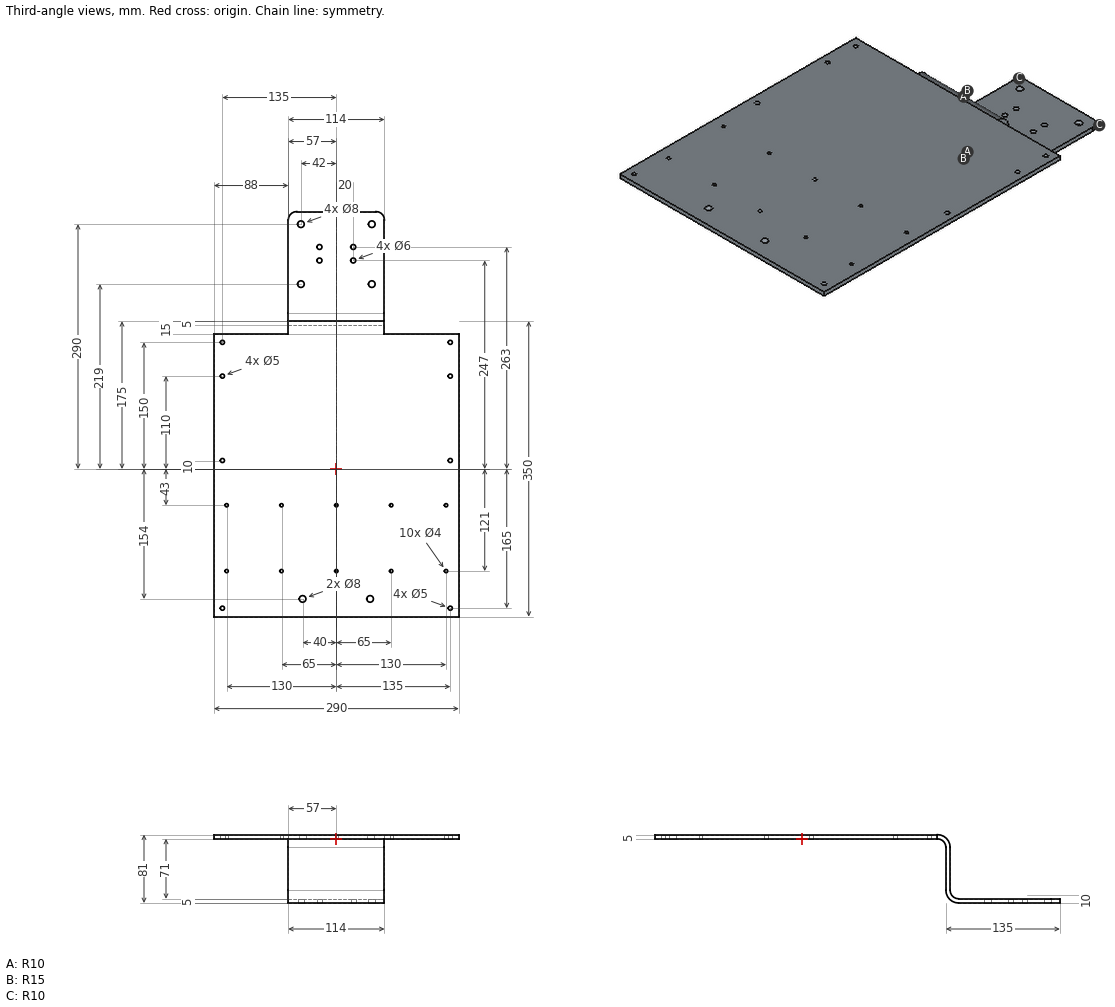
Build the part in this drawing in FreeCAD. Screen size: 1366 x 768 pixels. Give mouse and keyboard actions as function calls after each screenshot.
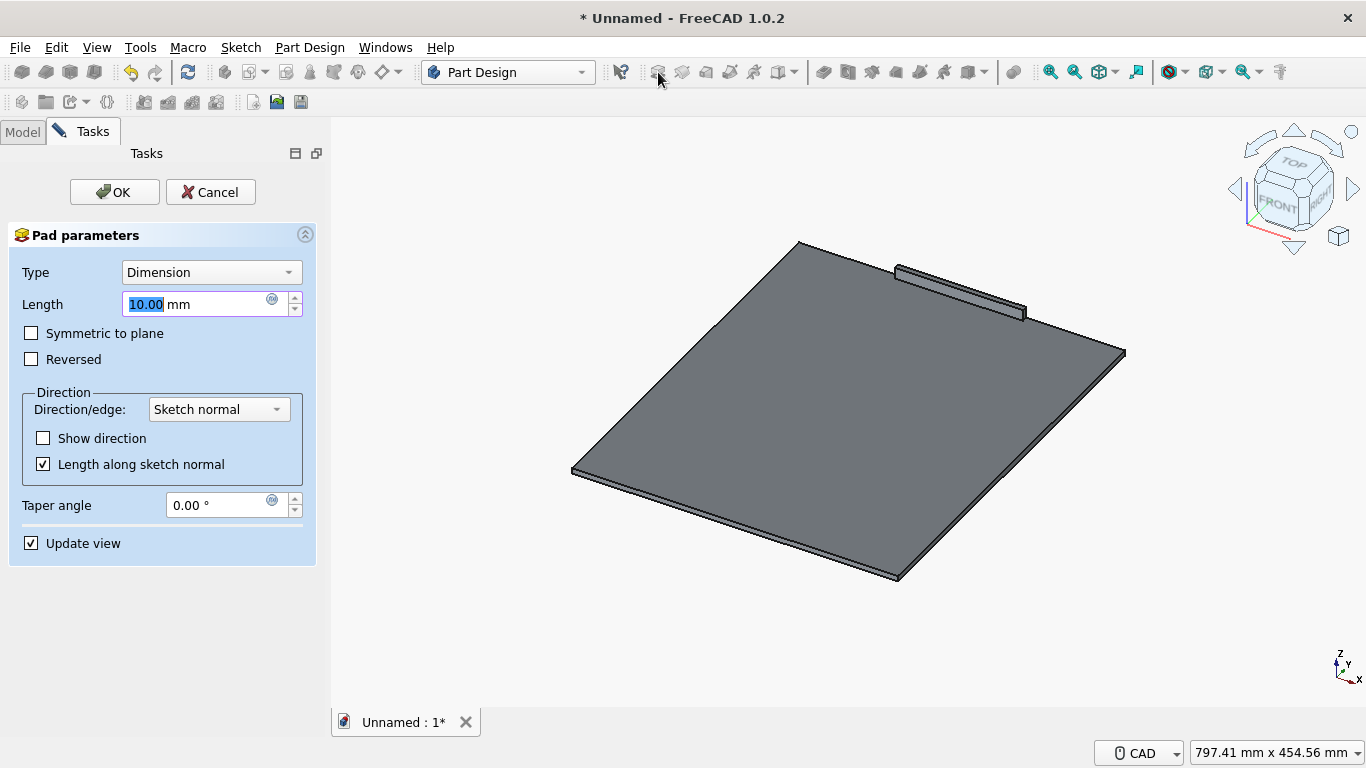
text(81)
key(Tab)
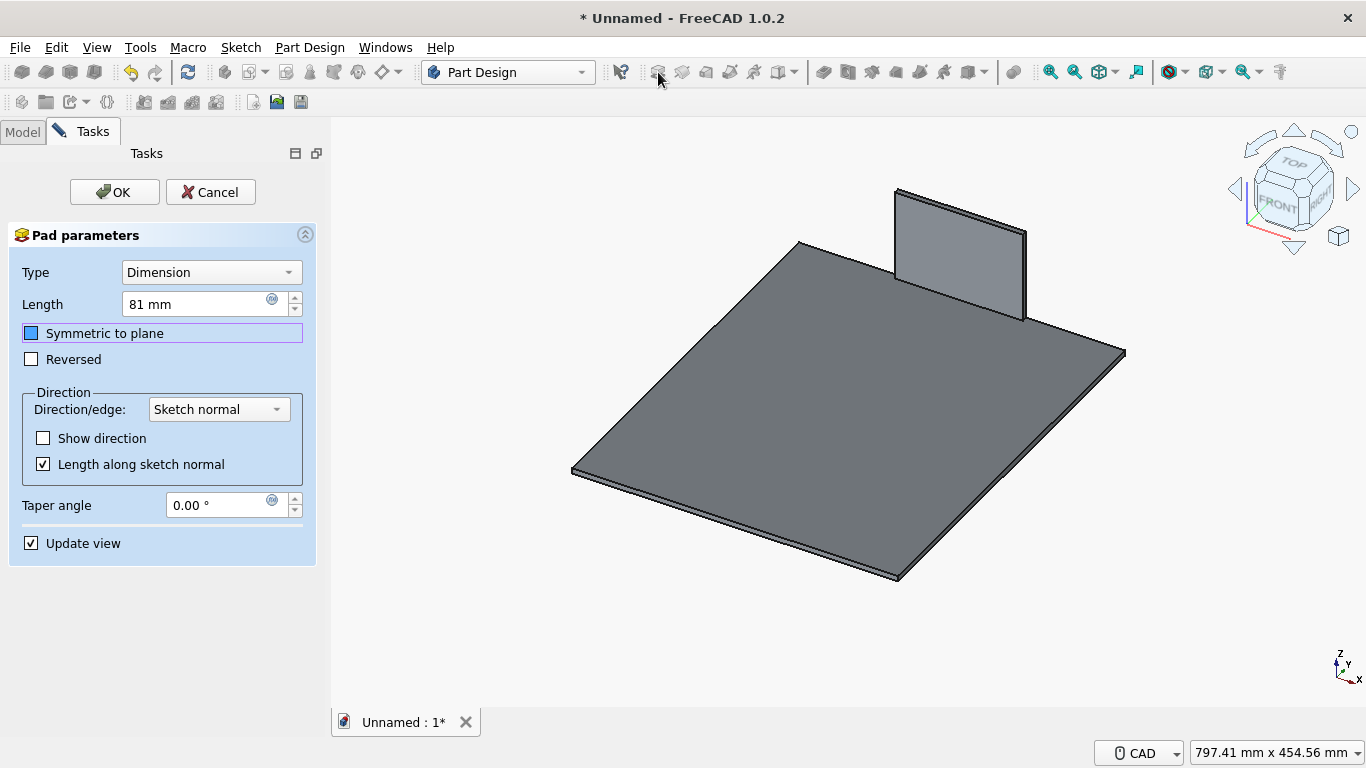
click(30, 359)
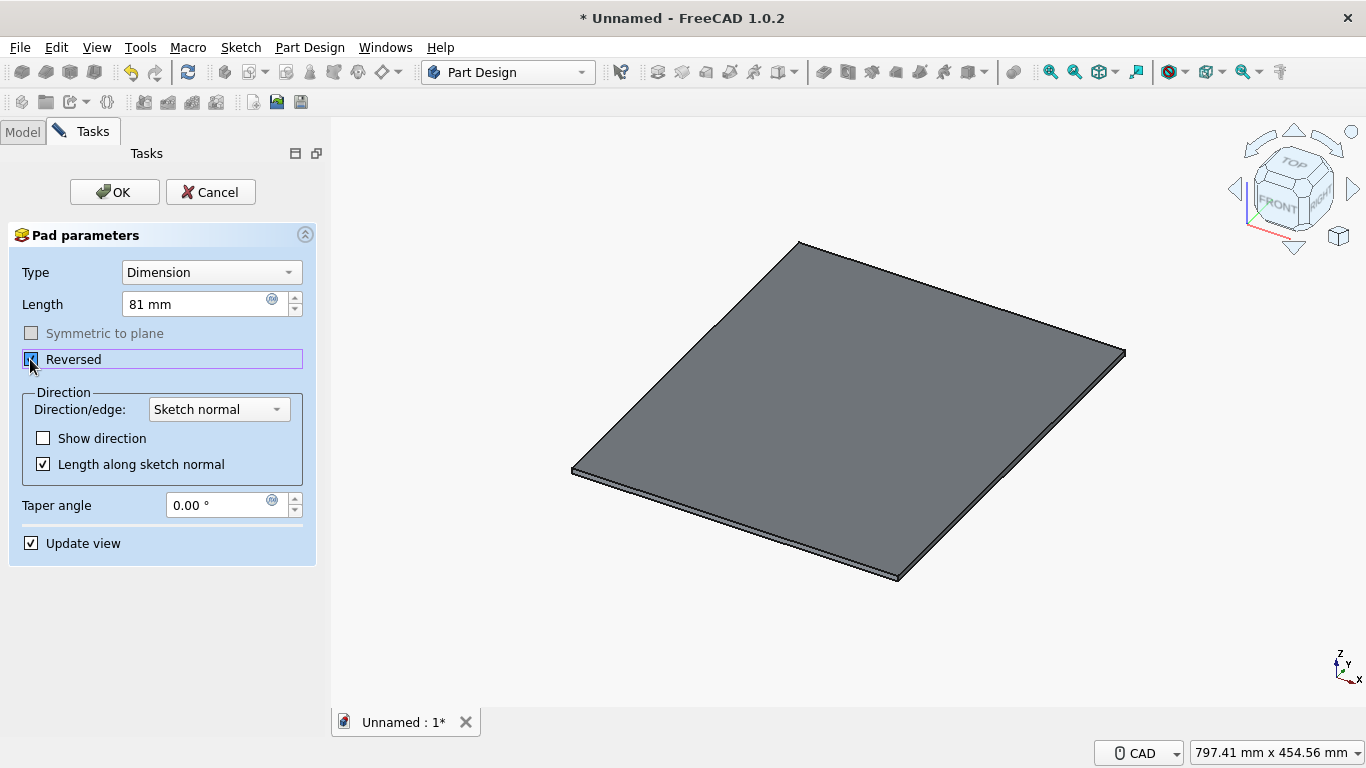
click(115, 192)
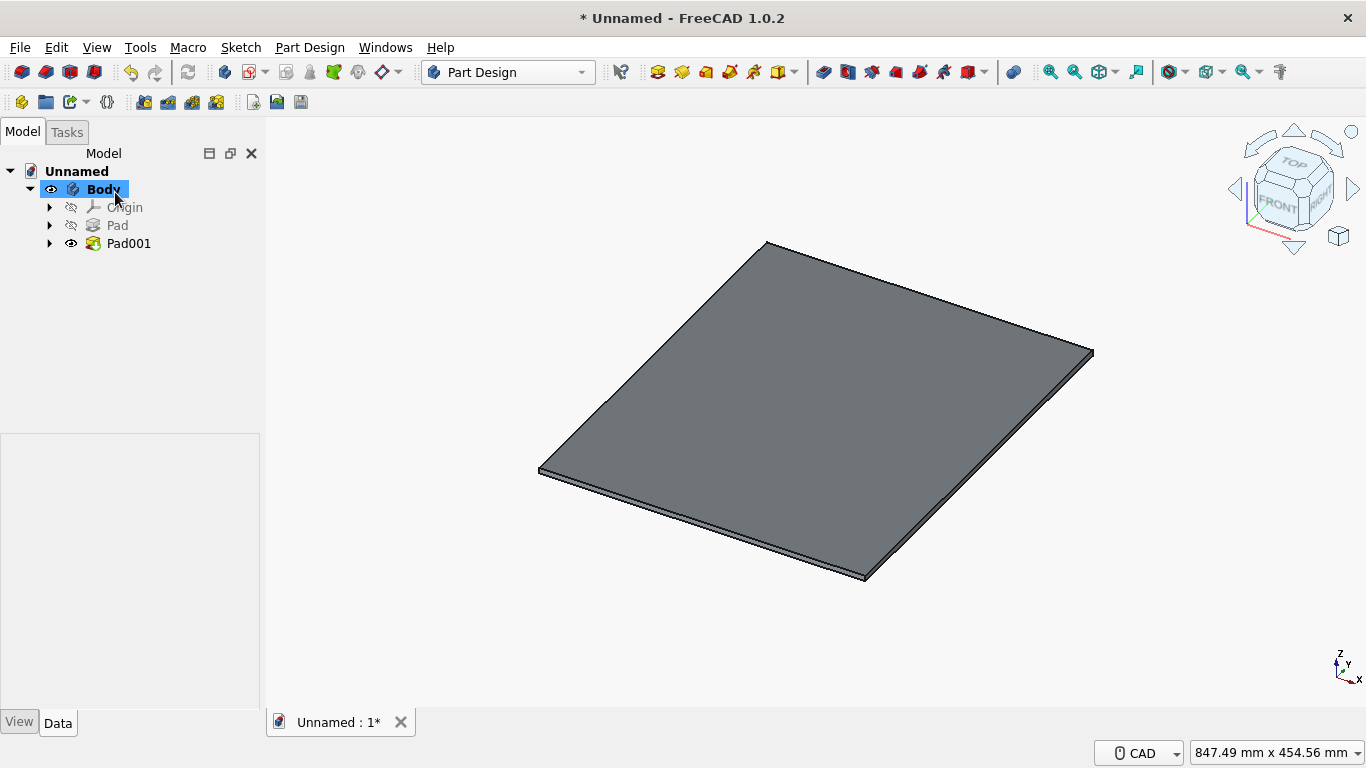
key(0)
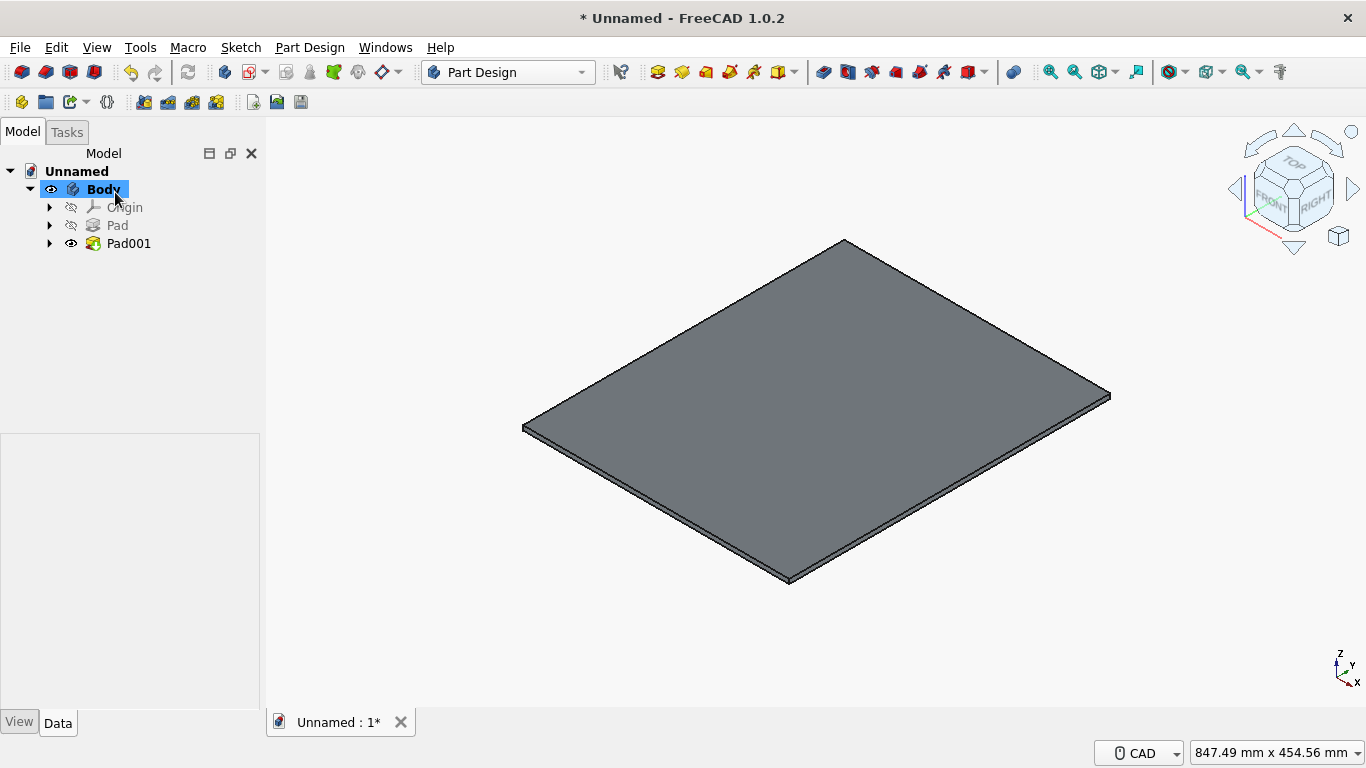
key(1)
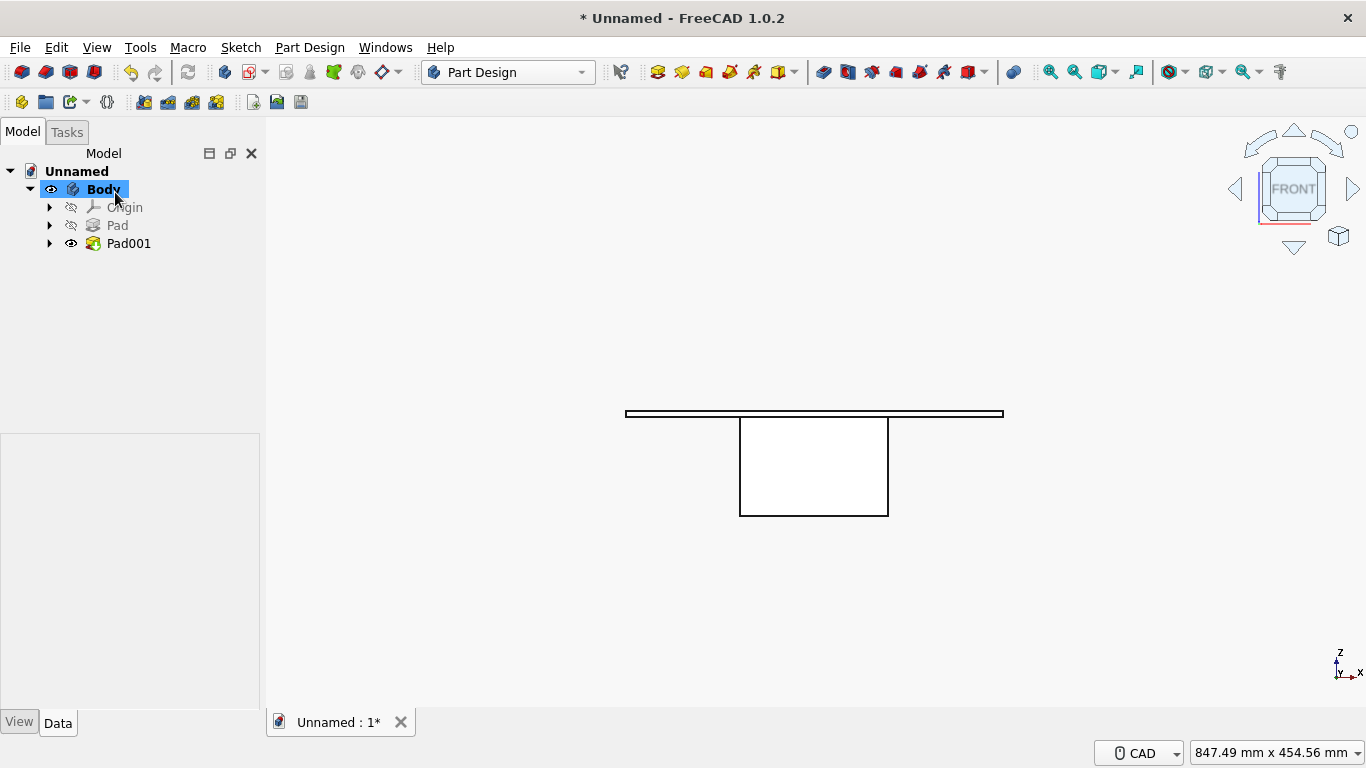
click(1052, 72)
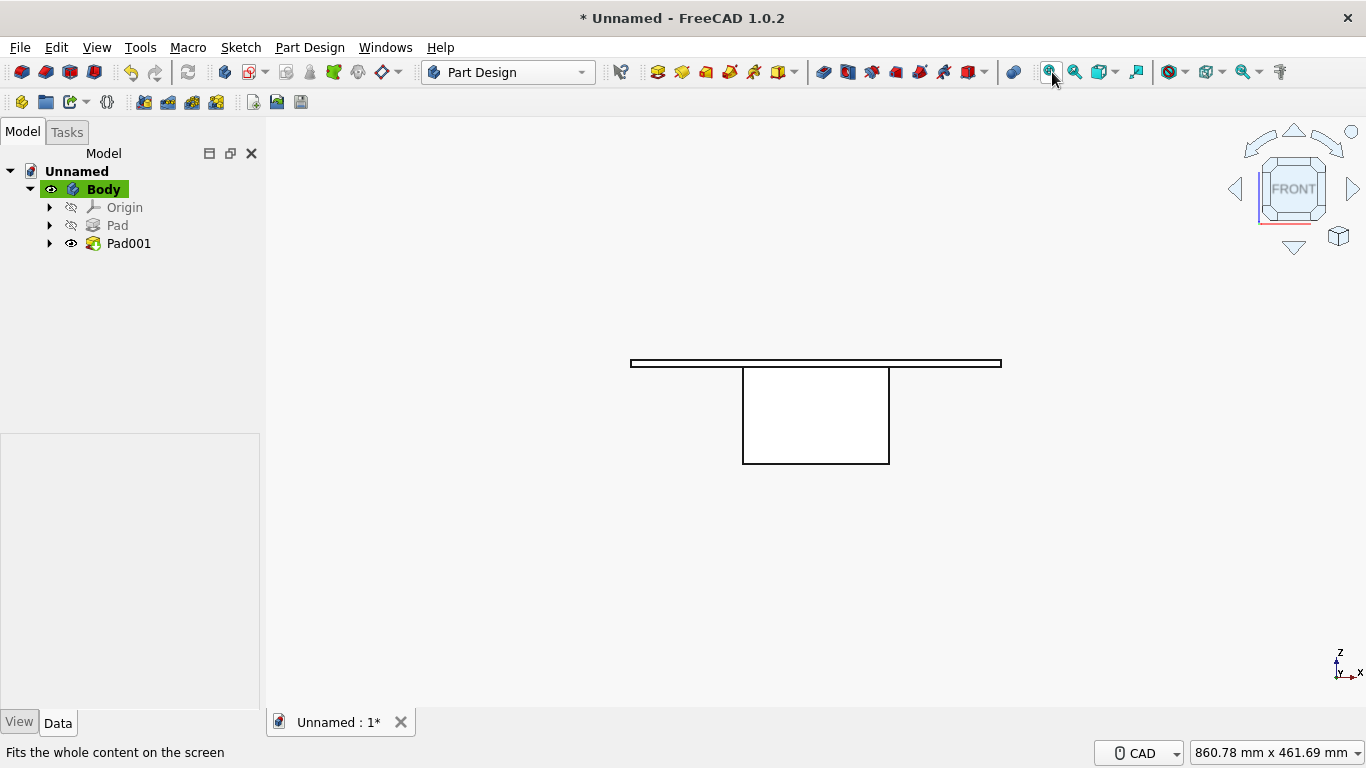
click(837, 414)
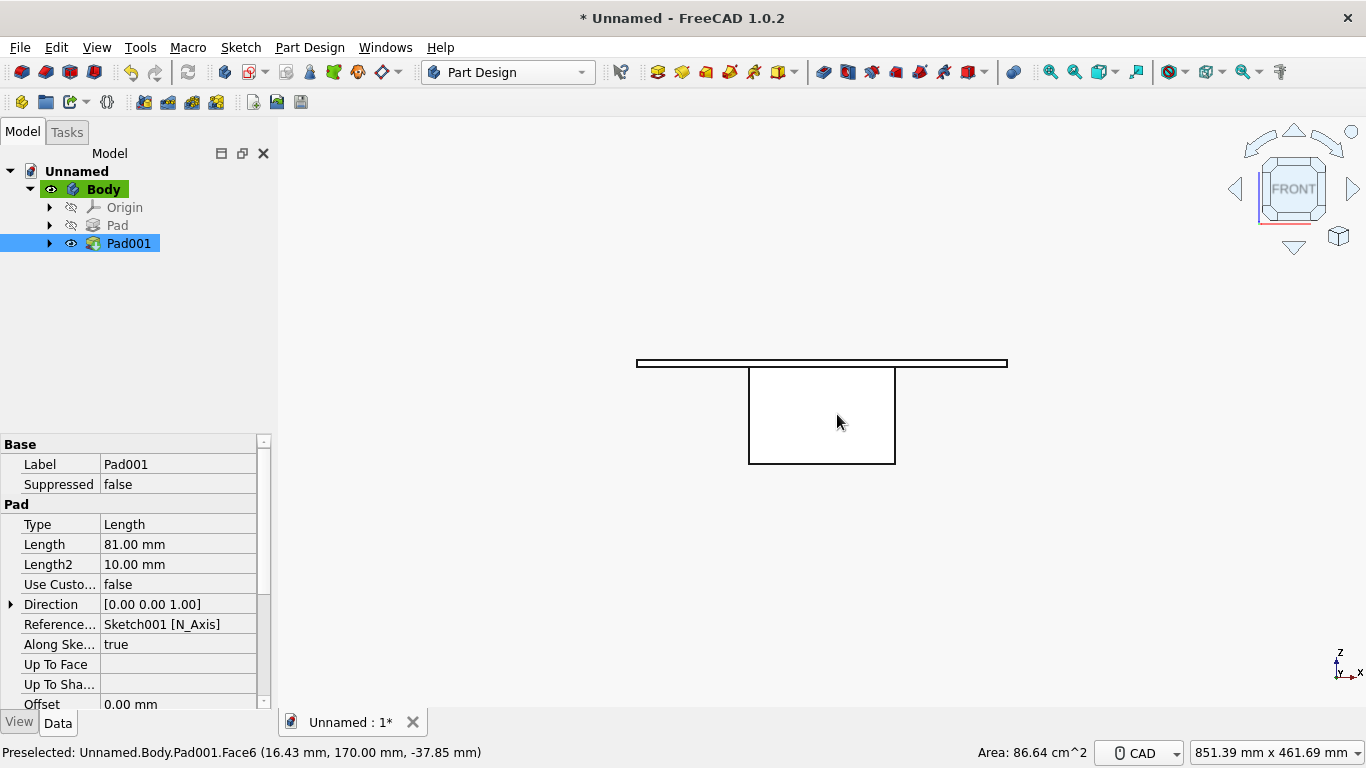
click(250, 72)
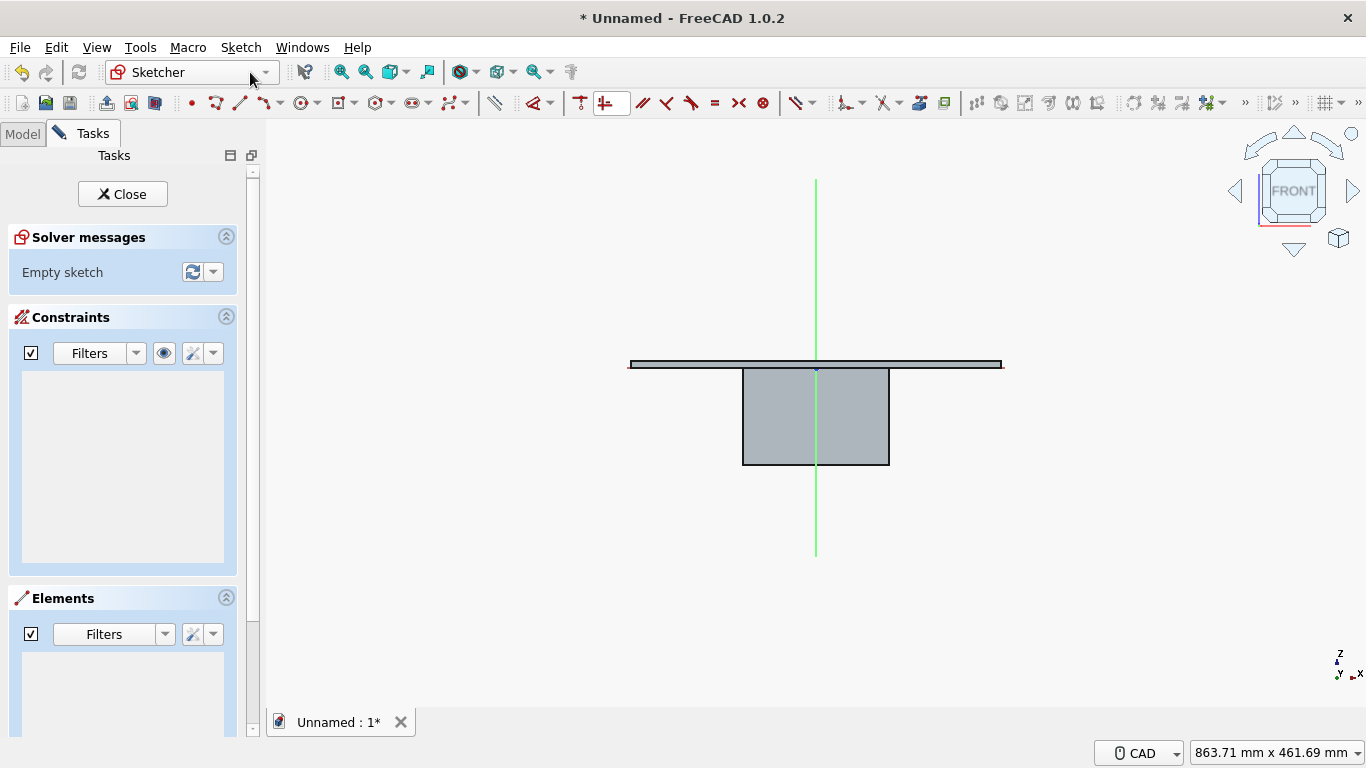
click(156, 104)